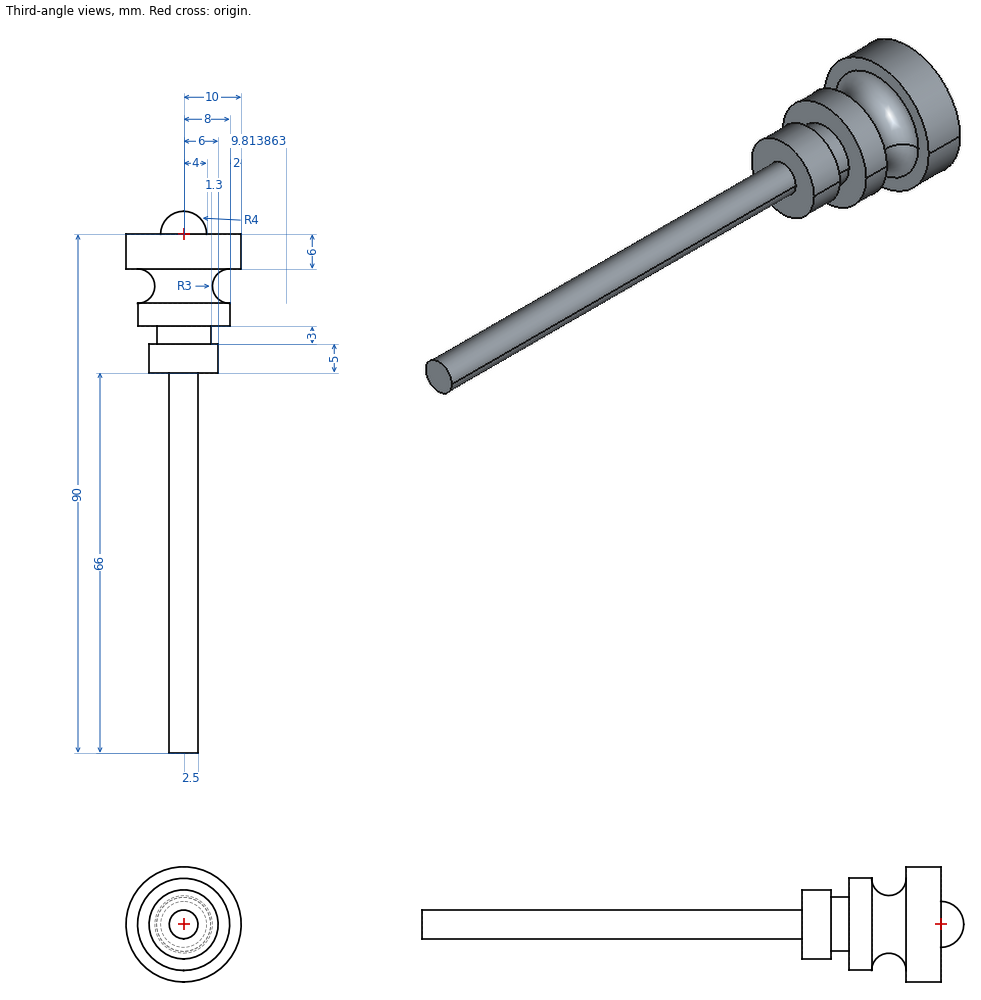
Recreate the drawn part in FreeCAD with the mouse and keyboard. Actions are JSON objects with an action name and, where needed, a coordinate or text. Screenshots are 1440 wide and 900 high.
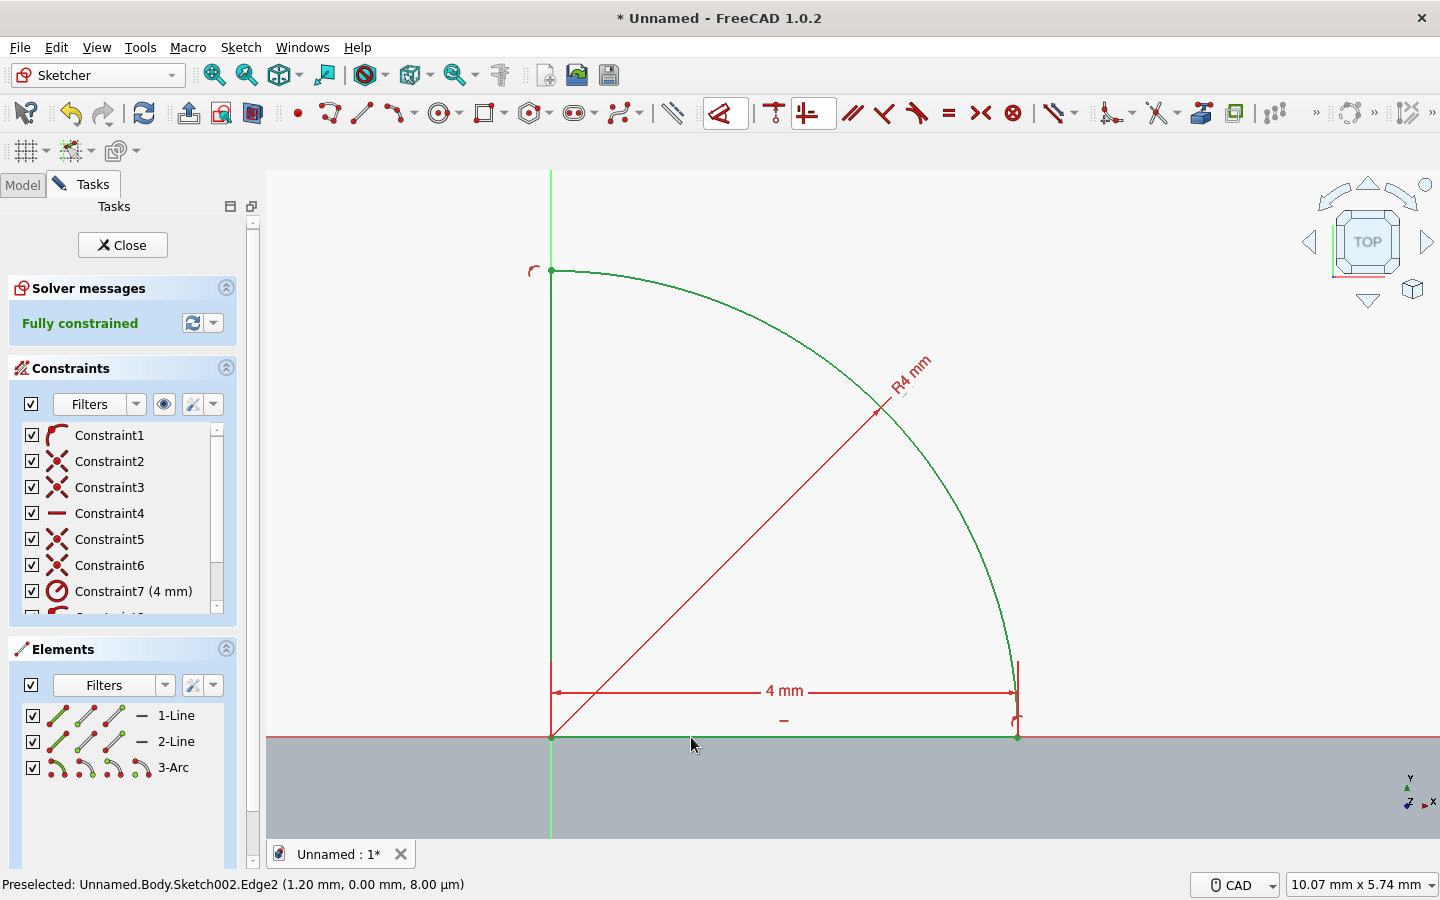
{"action": "left_click", "coordinate": [123, 245]}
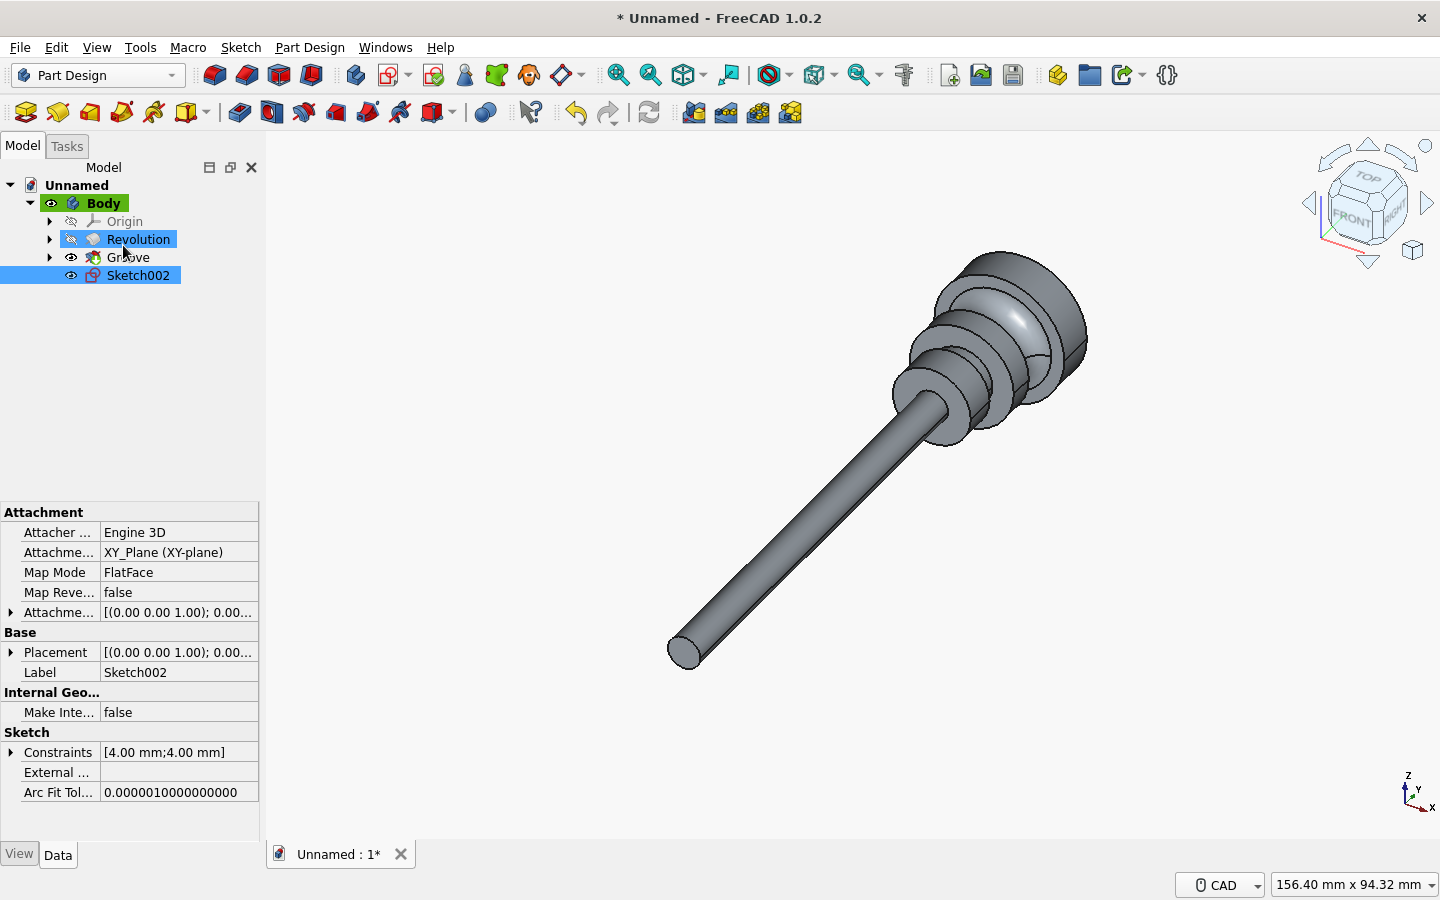
{"action": "left_click", "coordinate": [58, 112]}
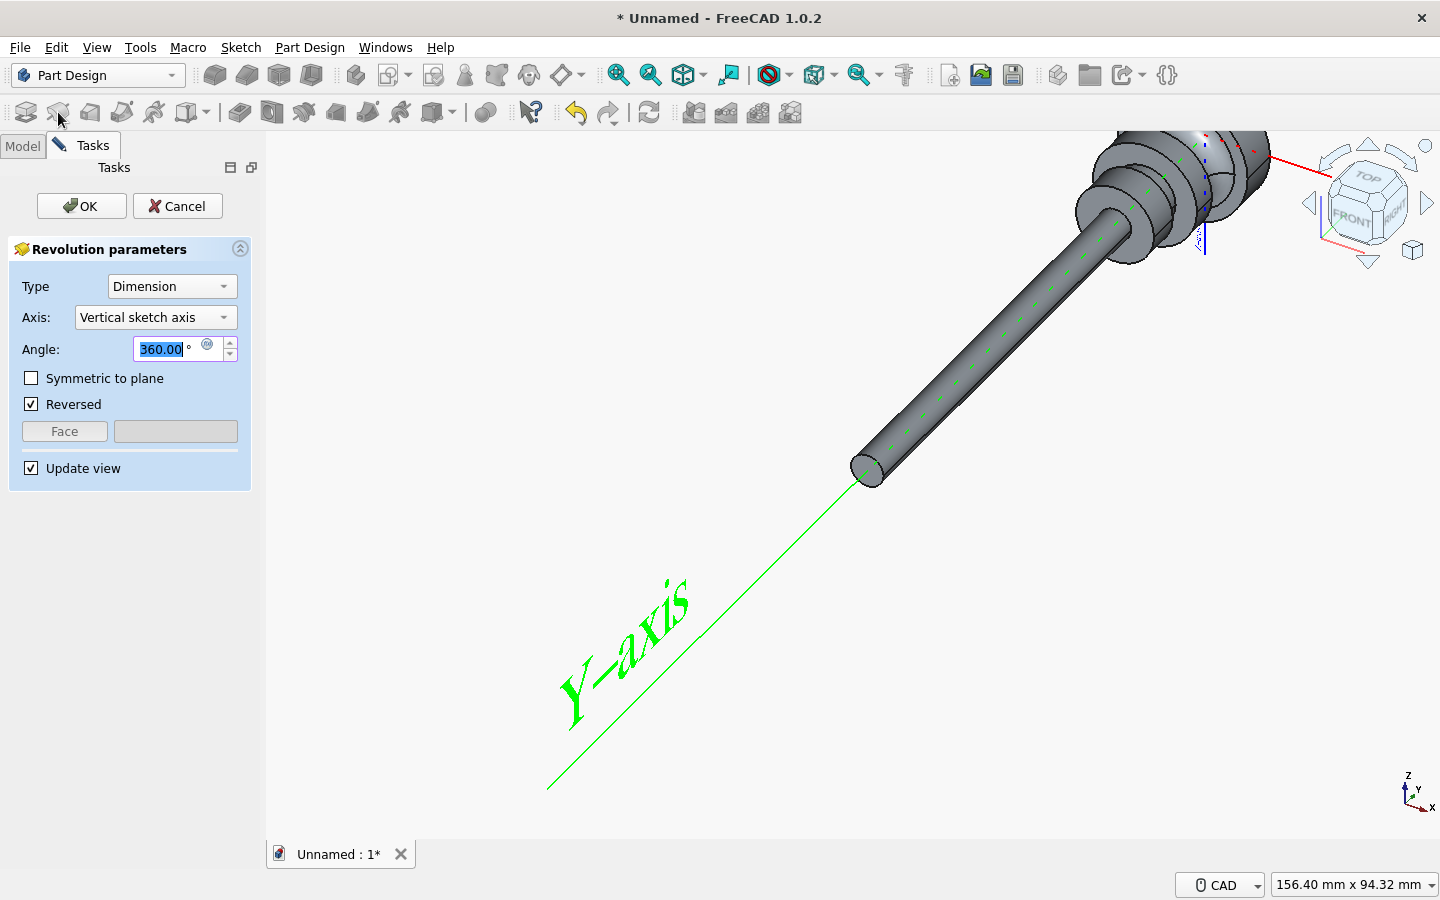
{"action": "left_click", "coordinate": [82, 206]}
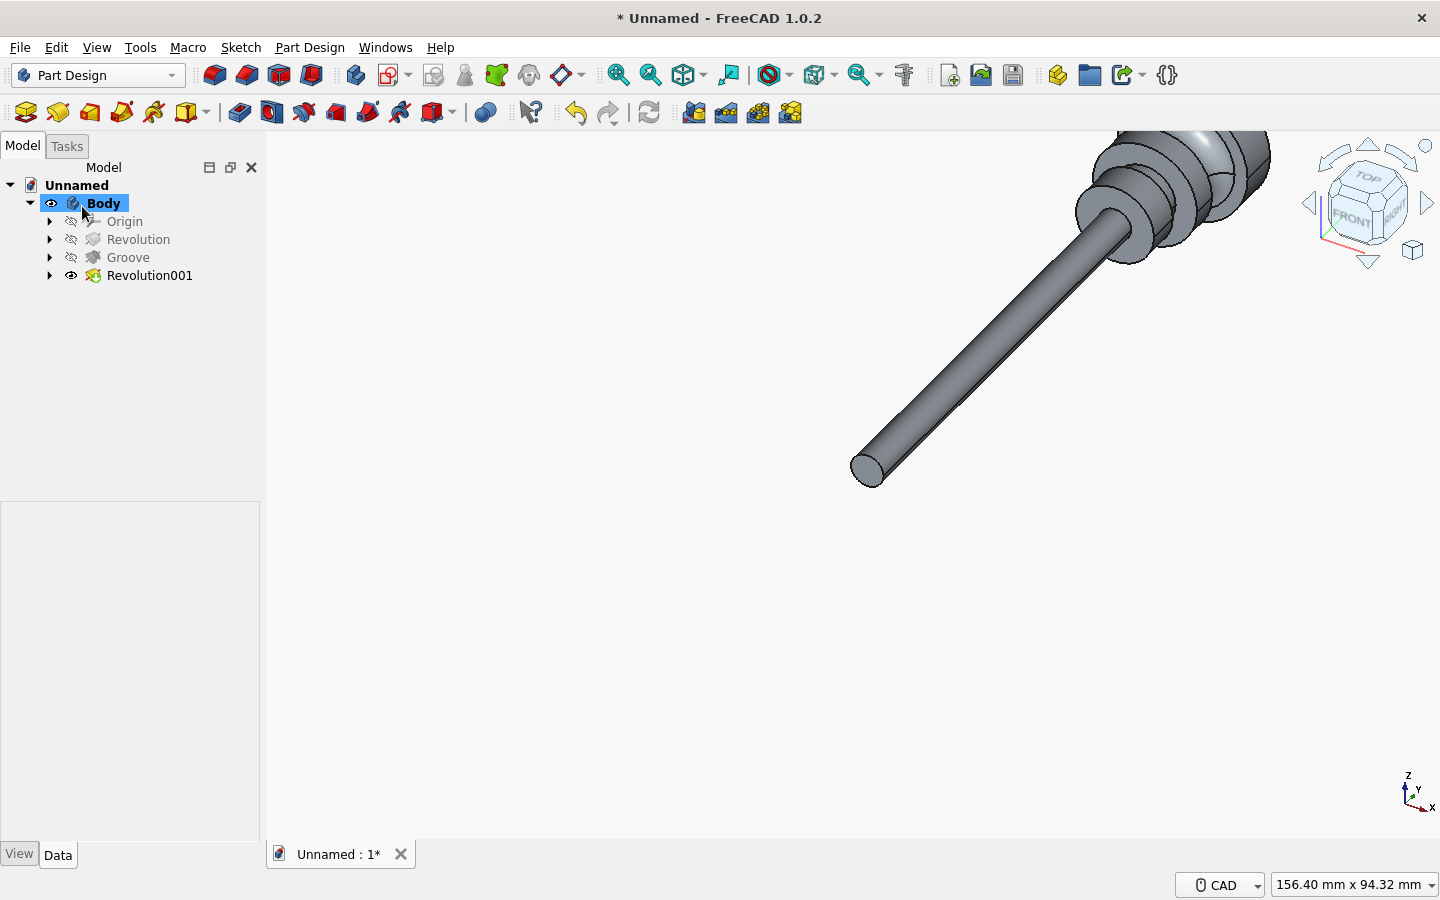
{"action": "key", "text": "0"}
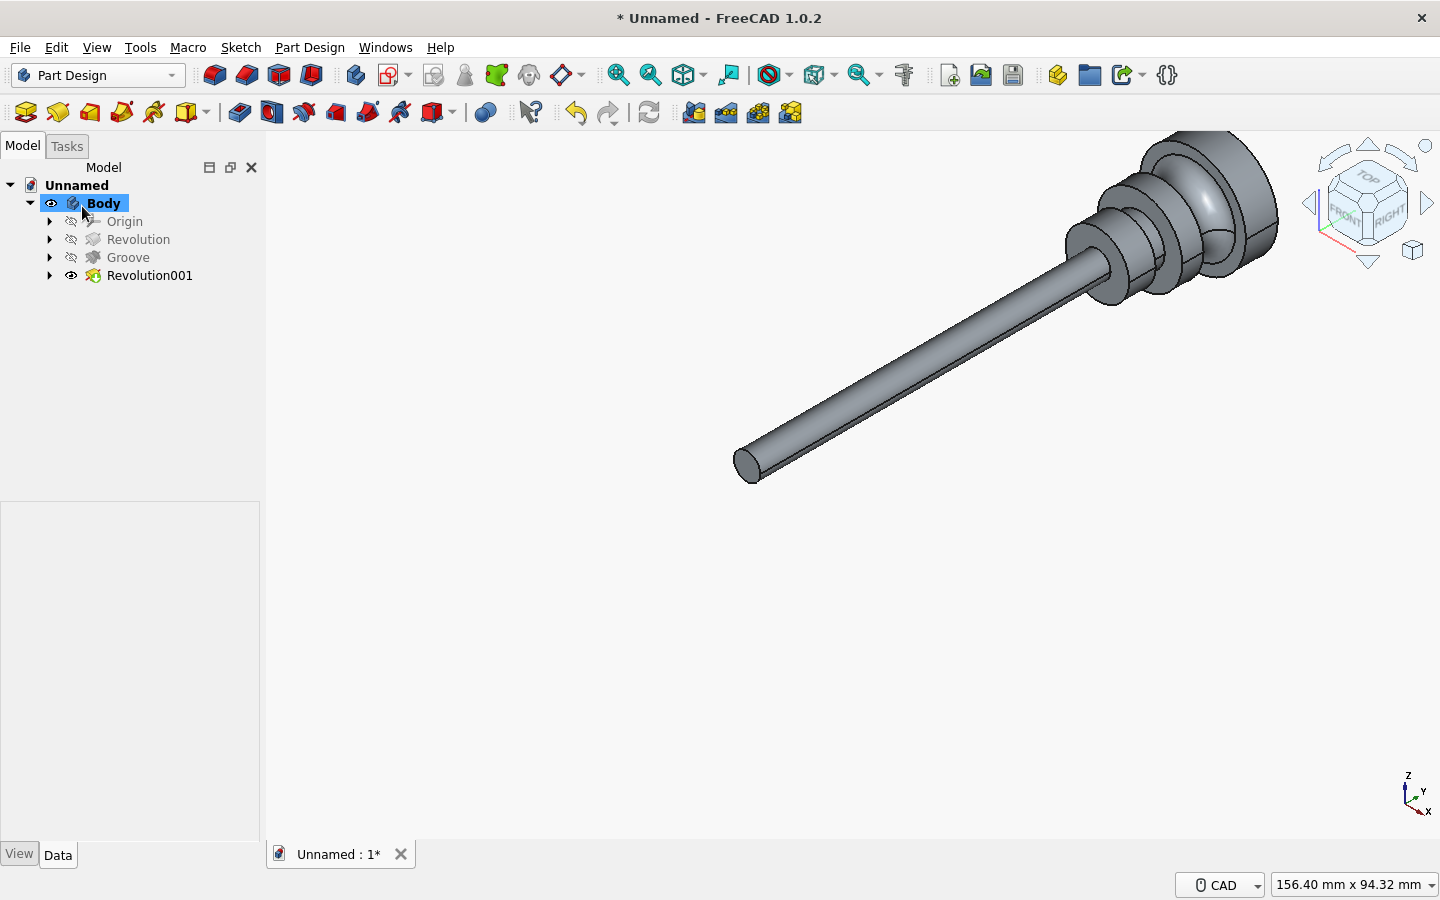
{"action": "left_click", "coordinate": [620, 76]}